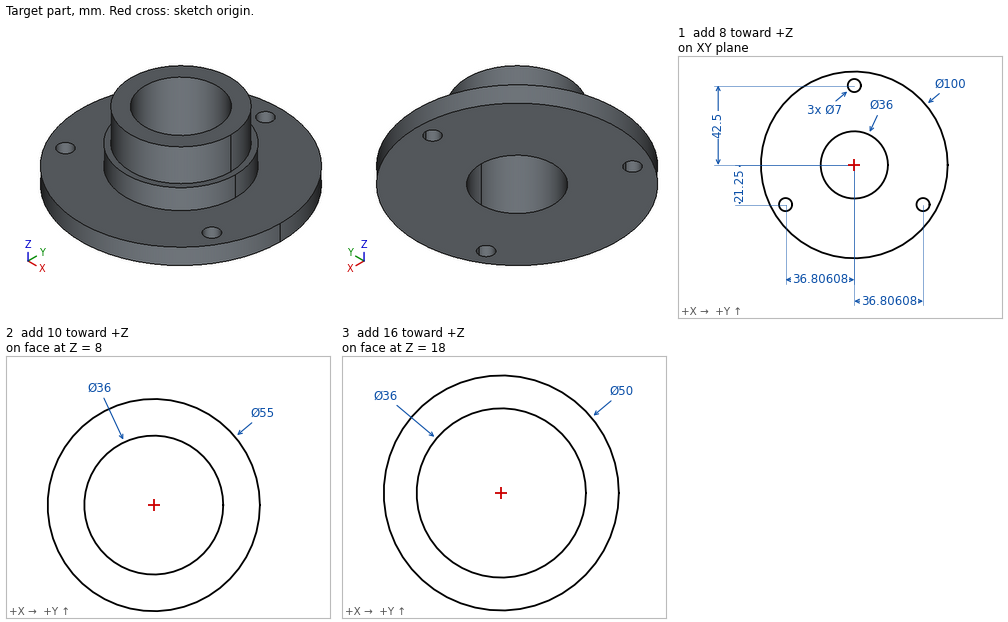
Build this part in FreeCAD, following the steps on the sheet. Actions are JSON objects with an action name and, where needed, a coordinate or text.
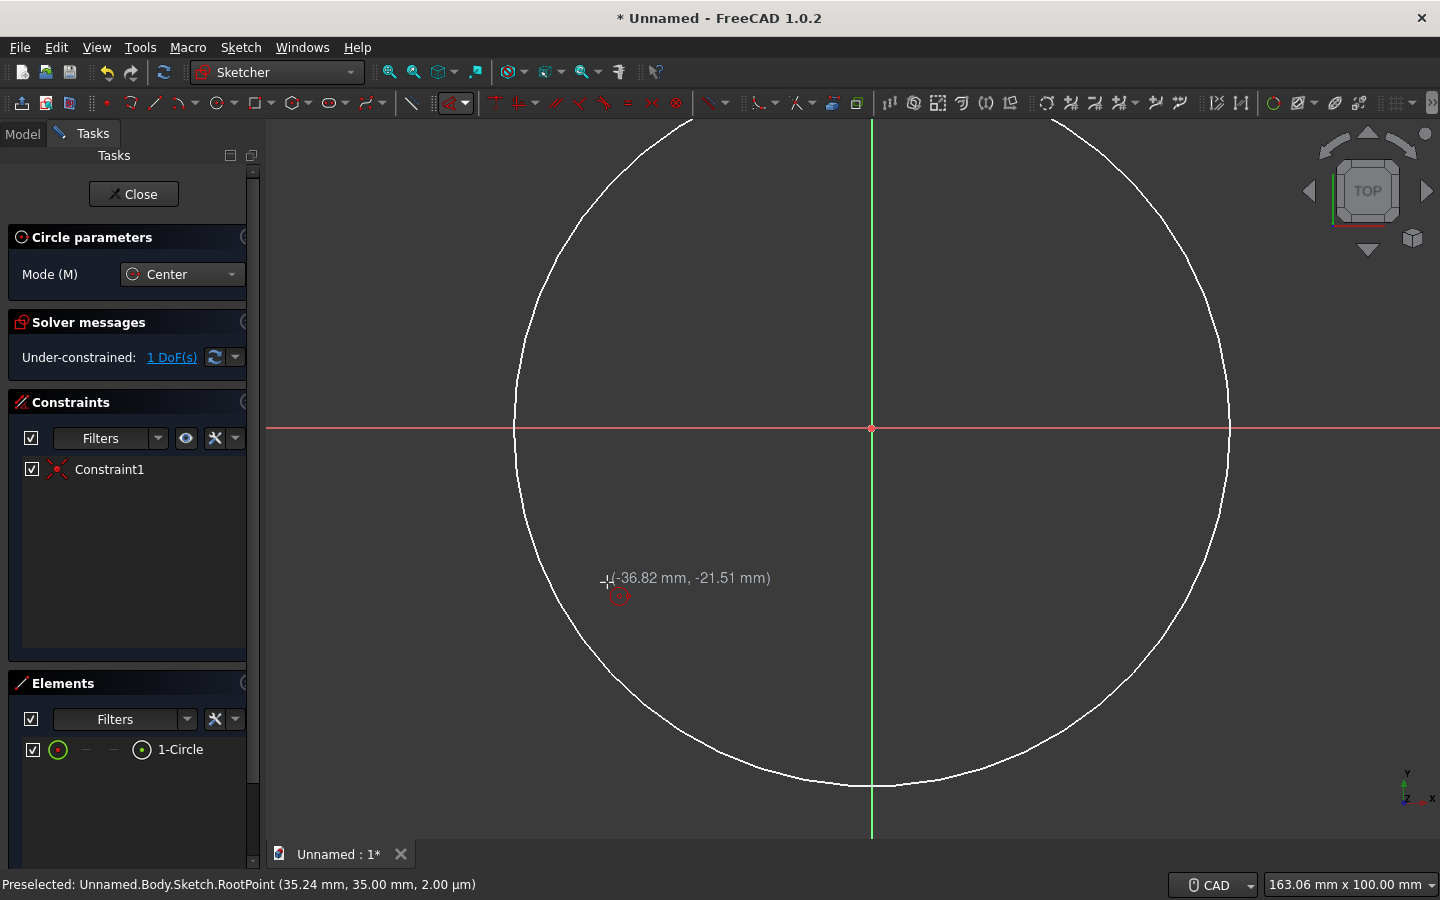
{"action": "left_click", "coordinate": [607, 581]}
{"action": "left_click", "coordinate": [625, 563]}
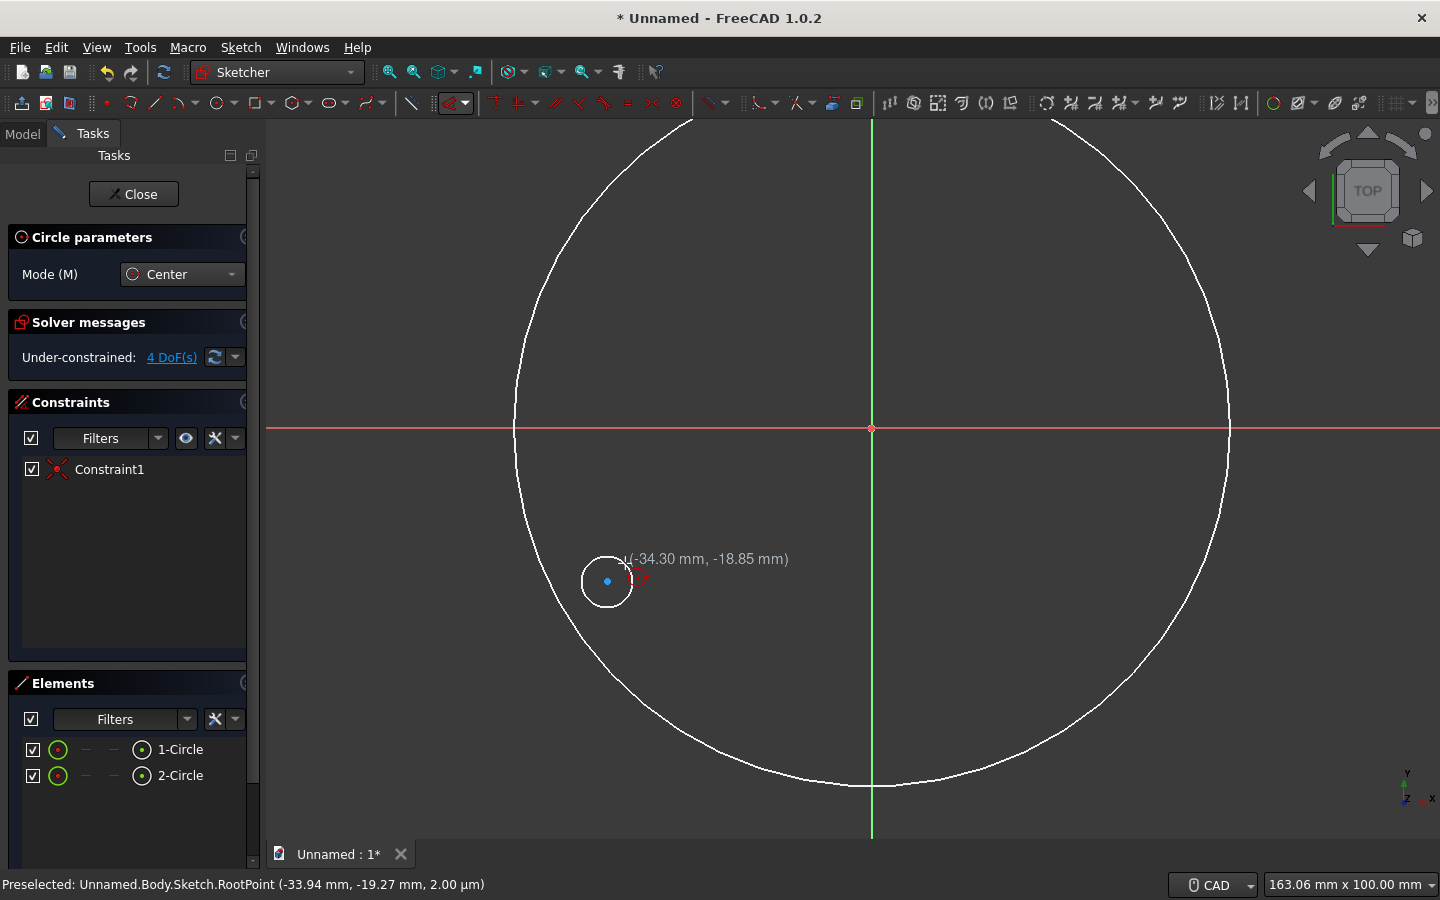
{"action": "left_click", "coordinate": [1137, 581]}
{"action": "left_click", "coordinate": [1155, 563]}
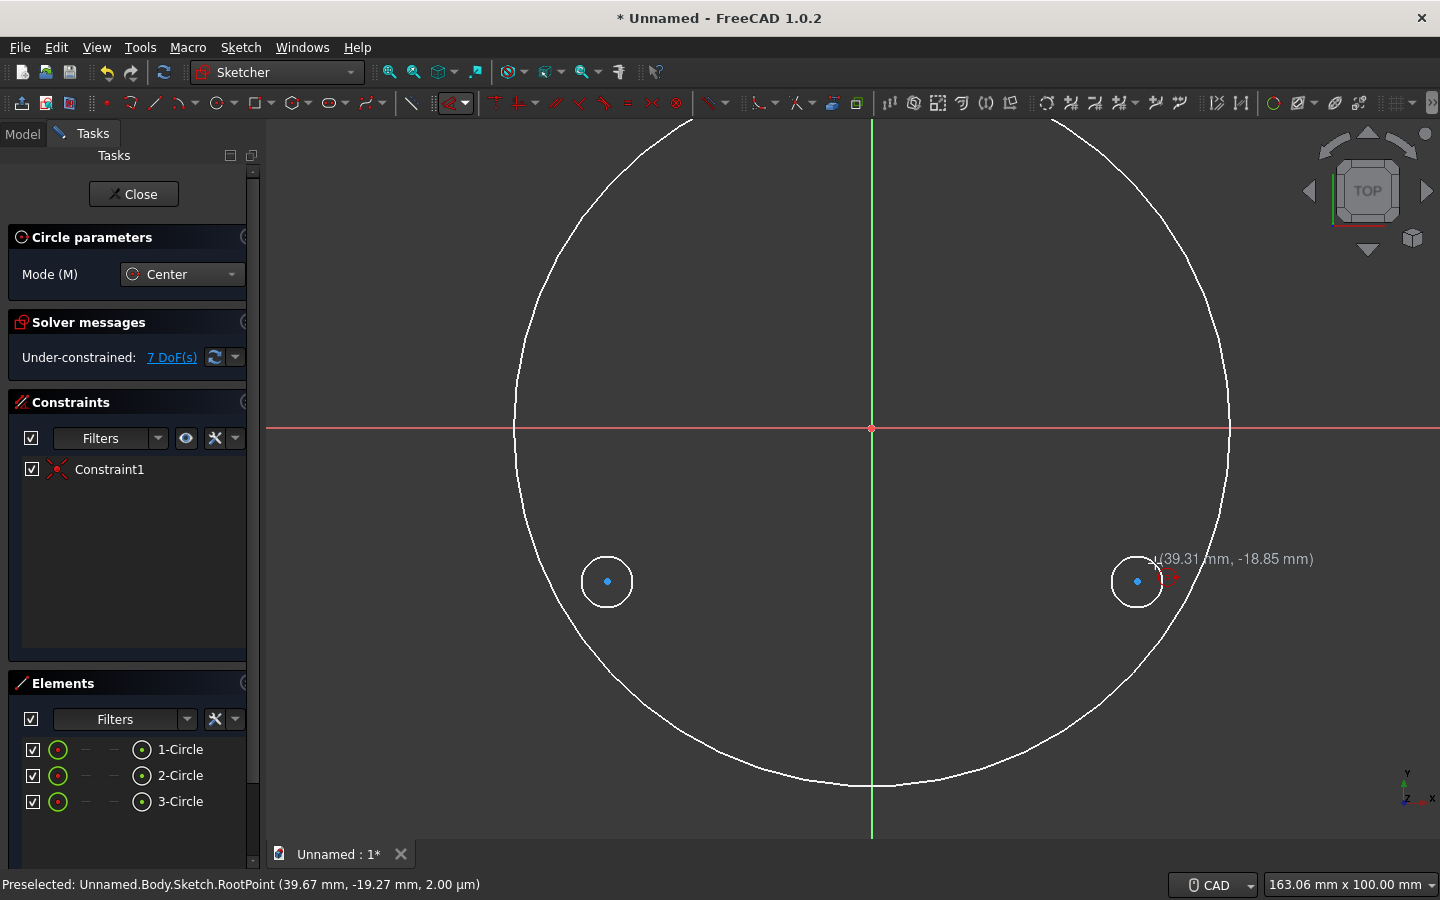
{"action": "left_click", "coordinate": [872, 428]}
{"action": "left_click", "coordinate": [964, 337]}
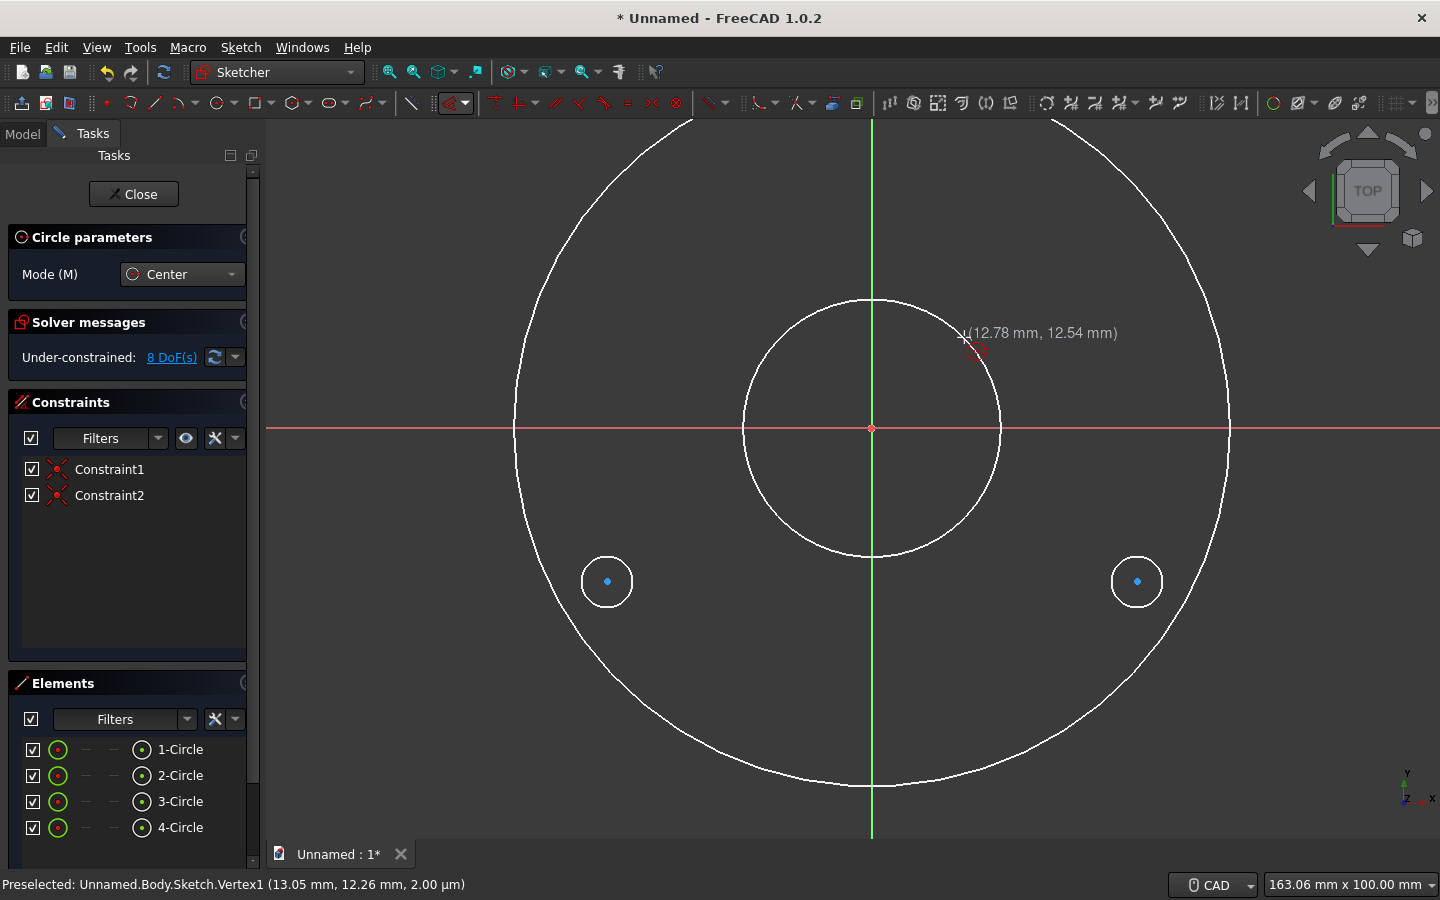
{"action": "scroll", "coordinate": [607, 582], "scroll_direction": "down", "scroll_amount": 2}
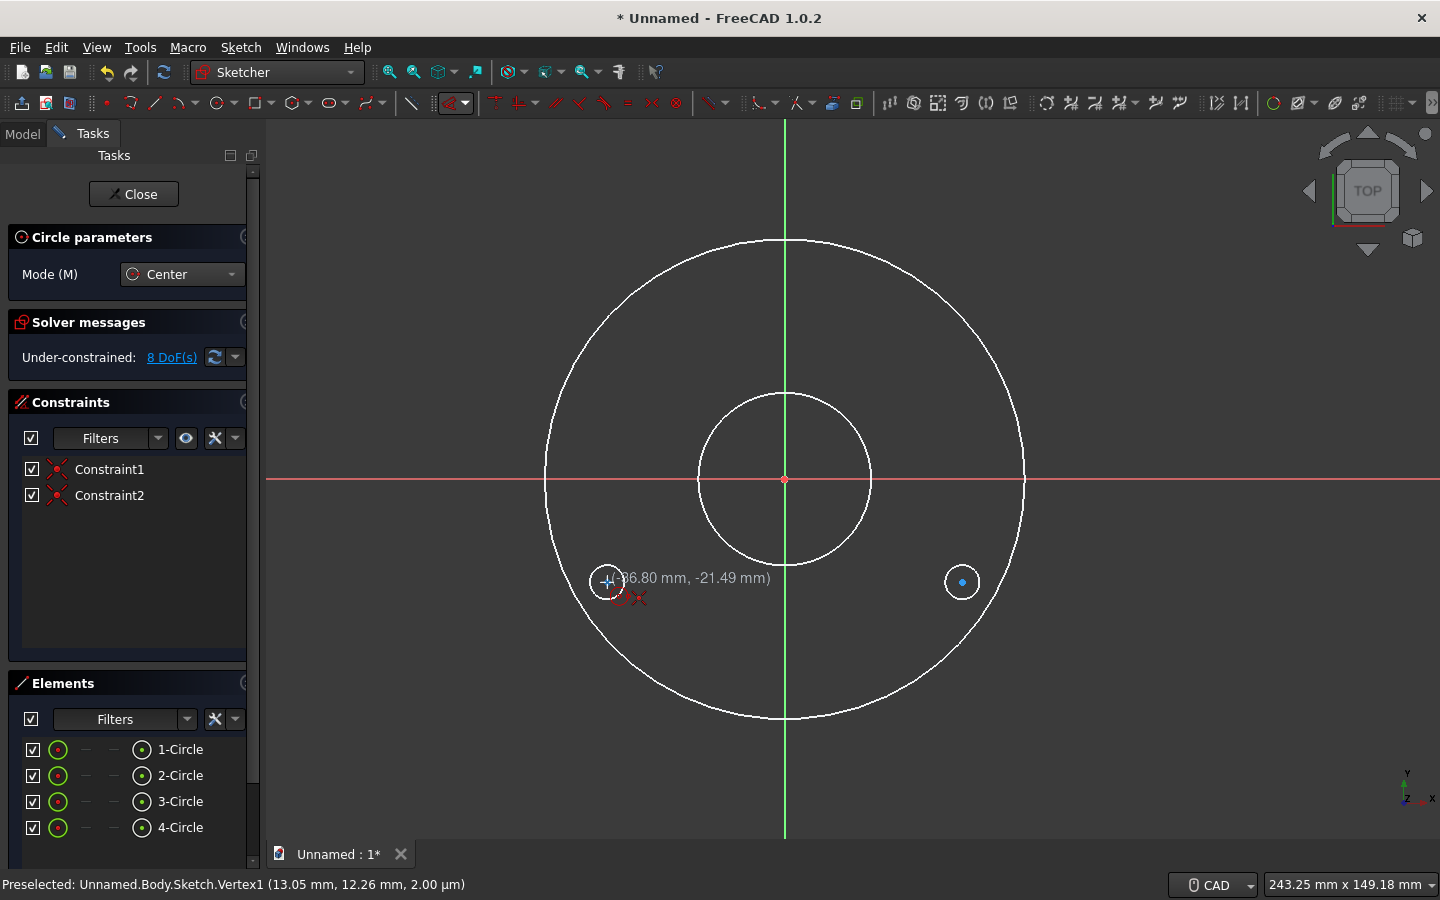
{"action": "scroll", "coordinate": [785, 274], "scroll_direction": "up", "scroll_amount": 2}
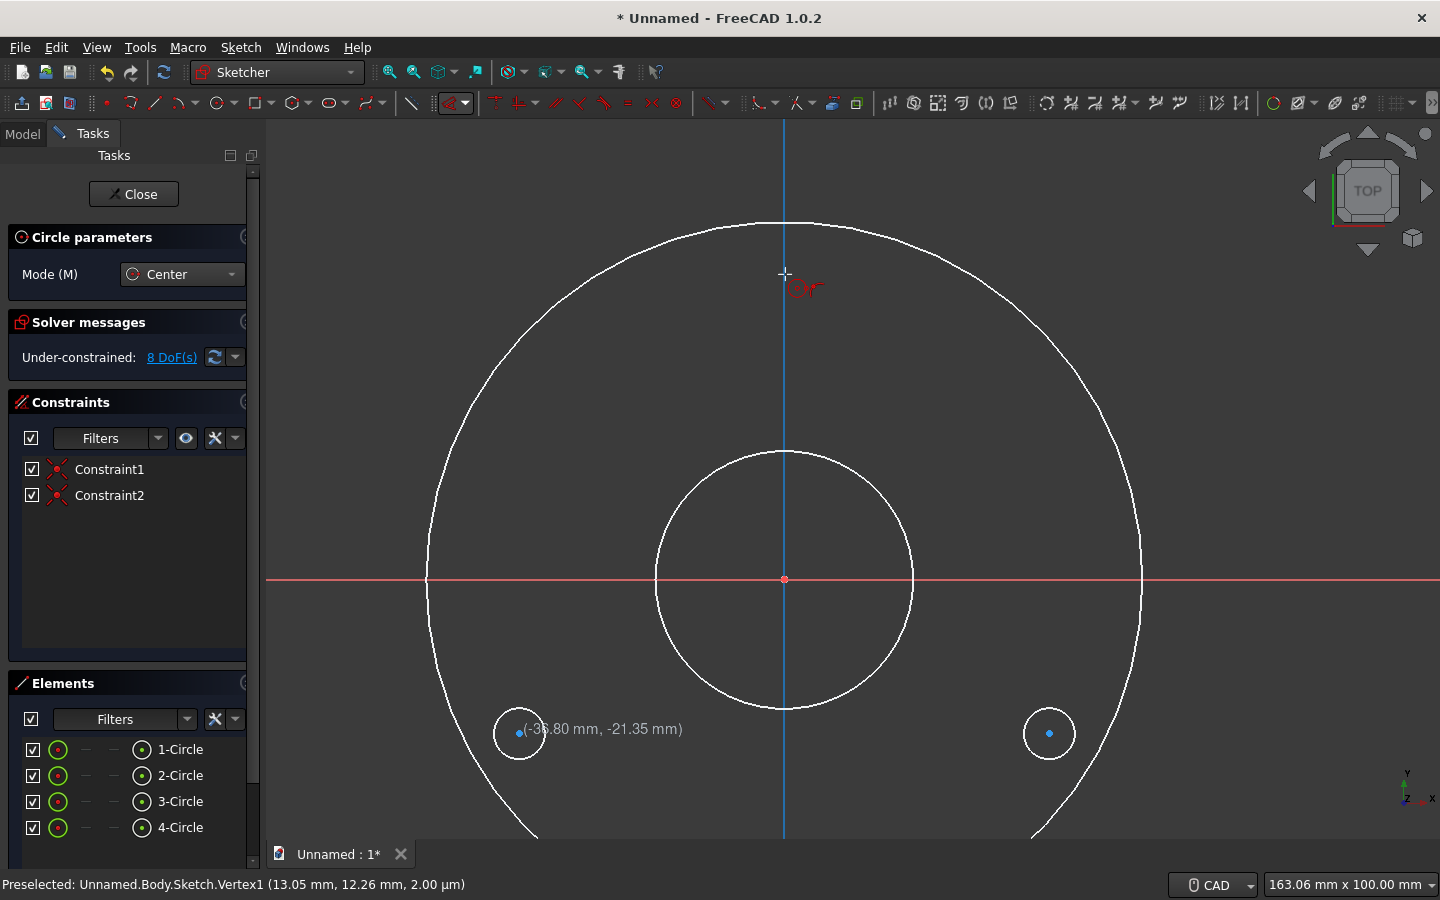
{"action": "left_click", "coordinate": [784, 274]}
{"action": "left_click", "coordinate": [802, 256]}
{"action": "key", "text": "Escape"}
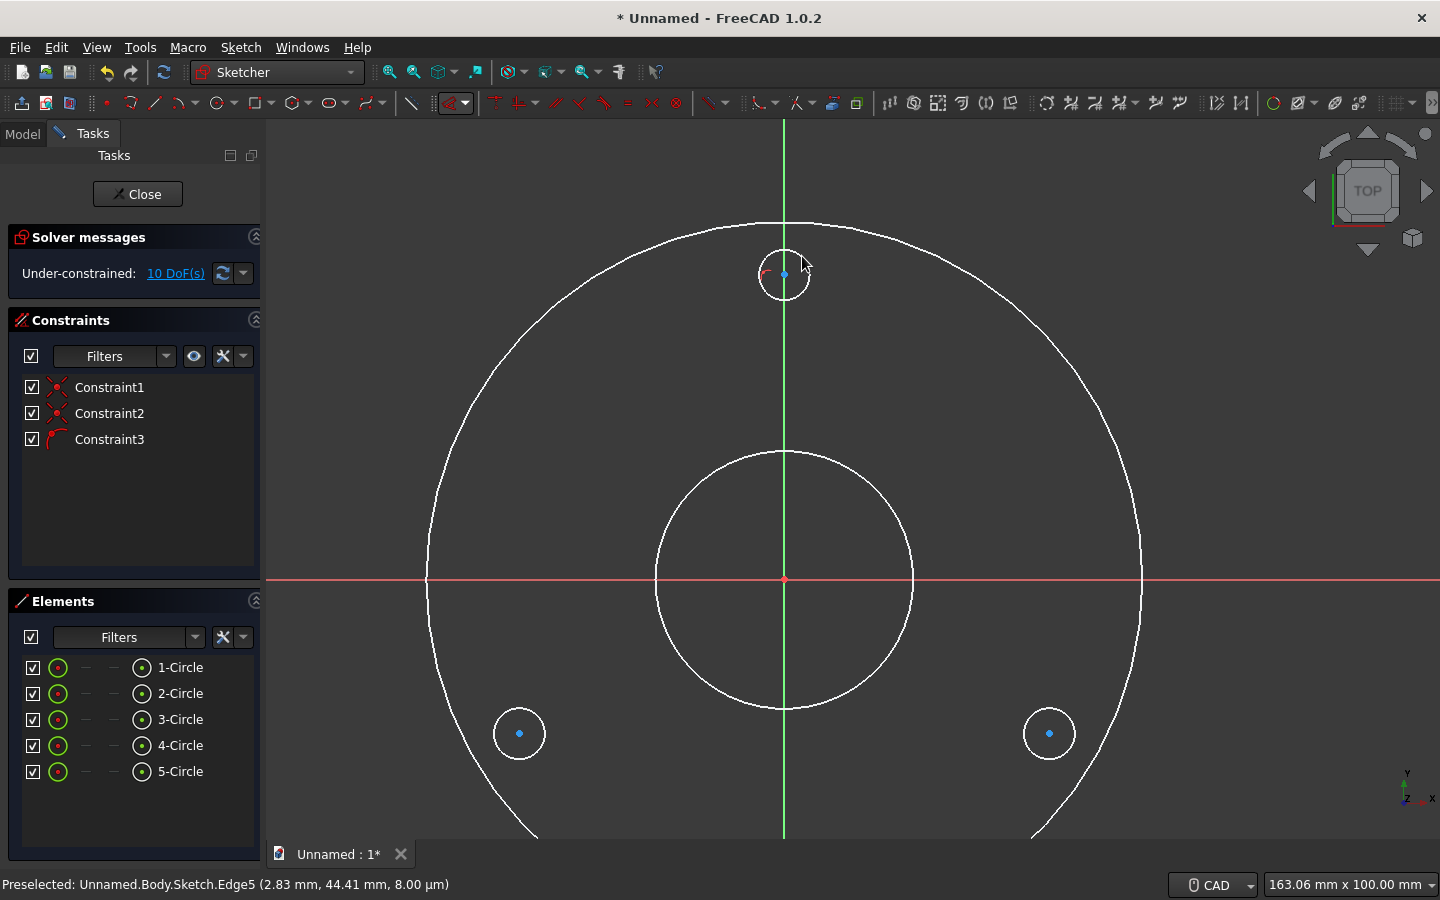
{"action": "left_click", "coordinate": [537, 716]}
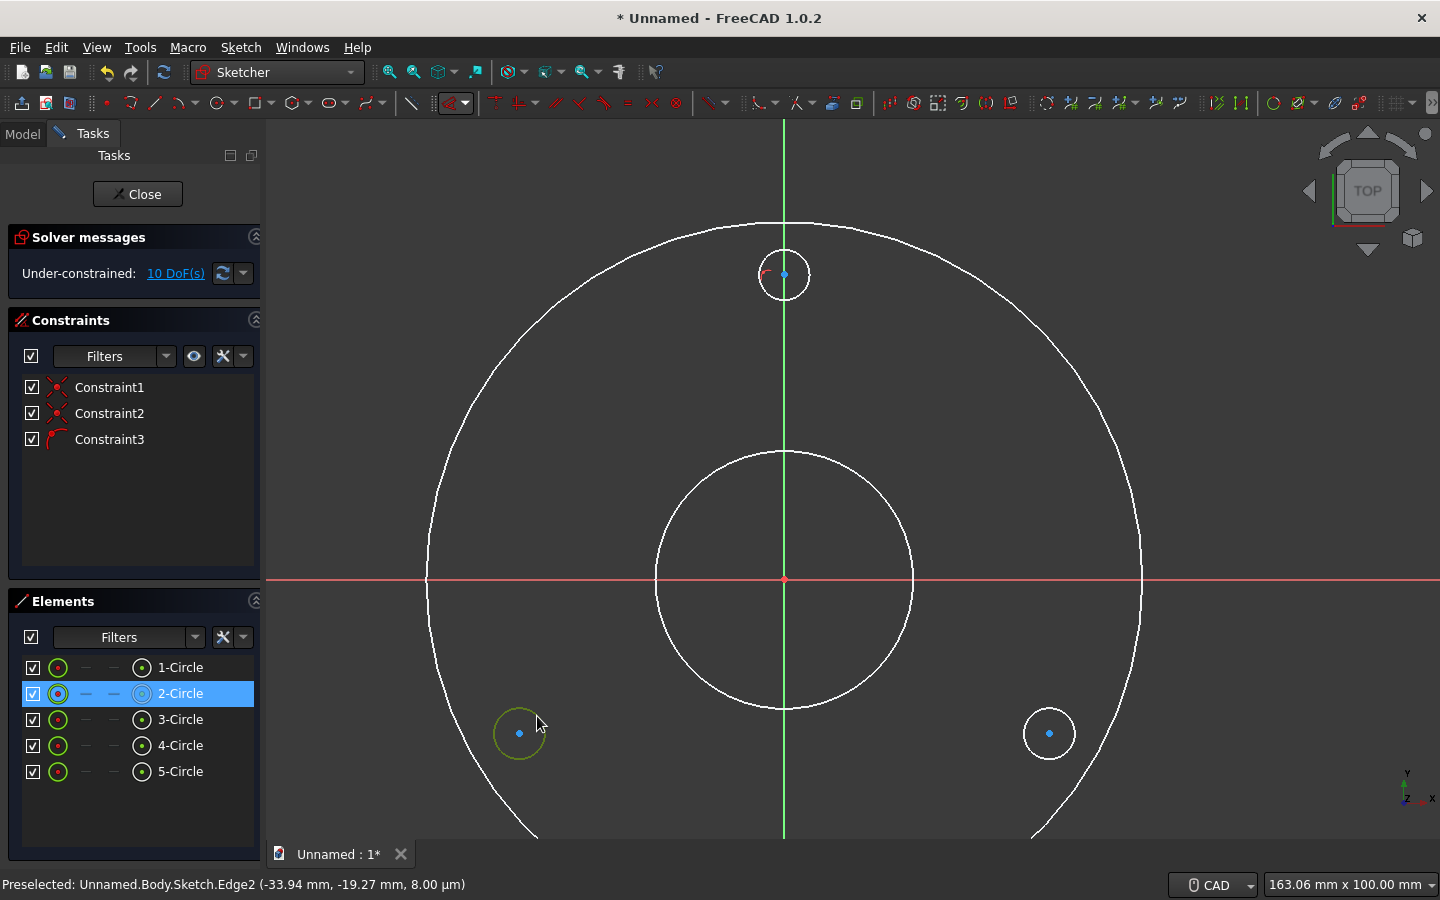
{"action": "left_click", "coordinate": [1067, 716]}